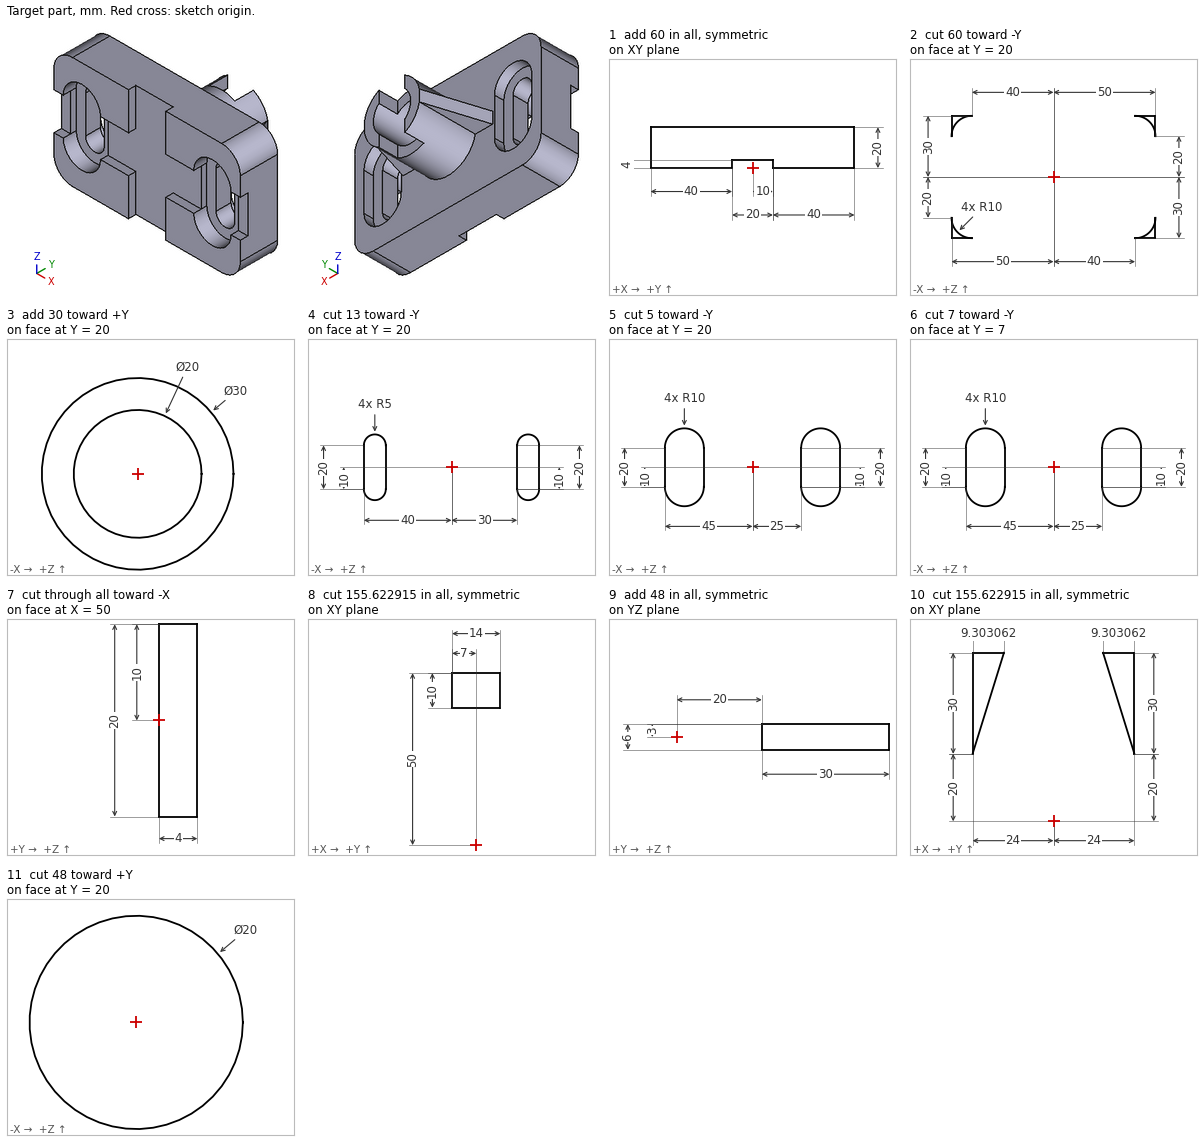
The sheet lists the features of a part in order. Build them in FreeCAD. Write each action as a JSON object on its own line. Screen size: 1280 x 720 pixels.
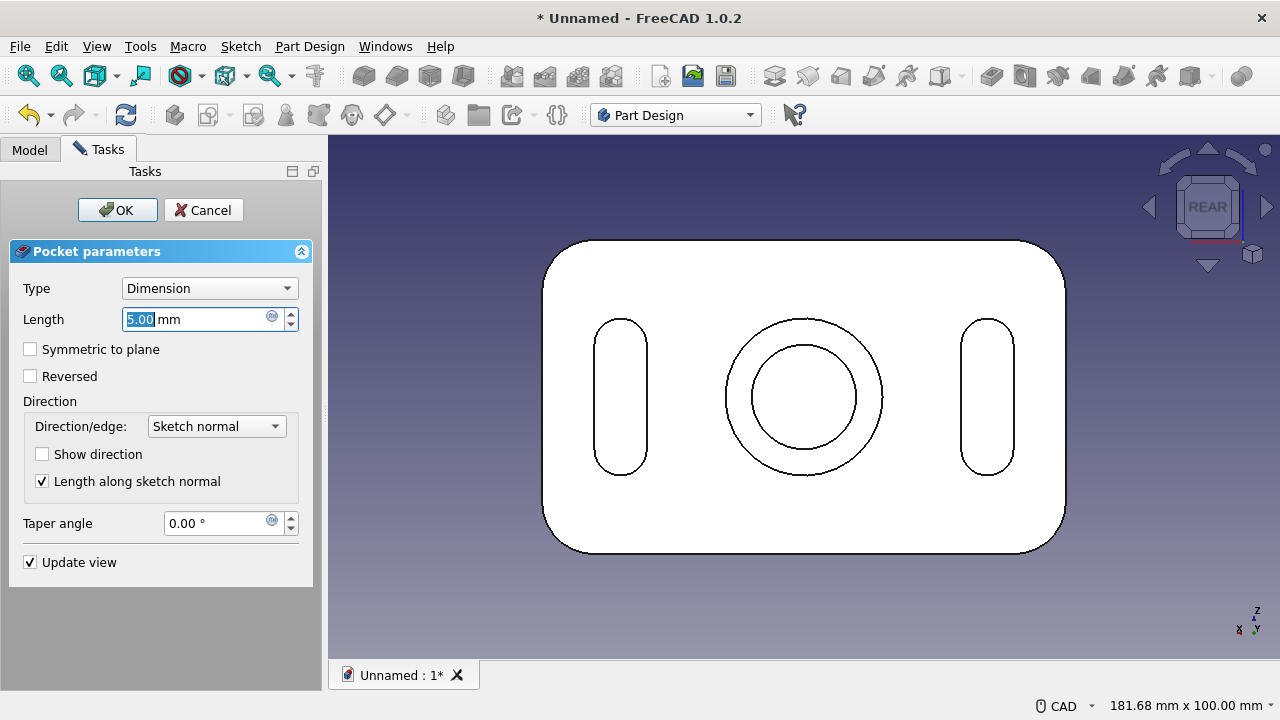
{"action": "type", "text": "13"}
{"action": "key", "text": "Tab"}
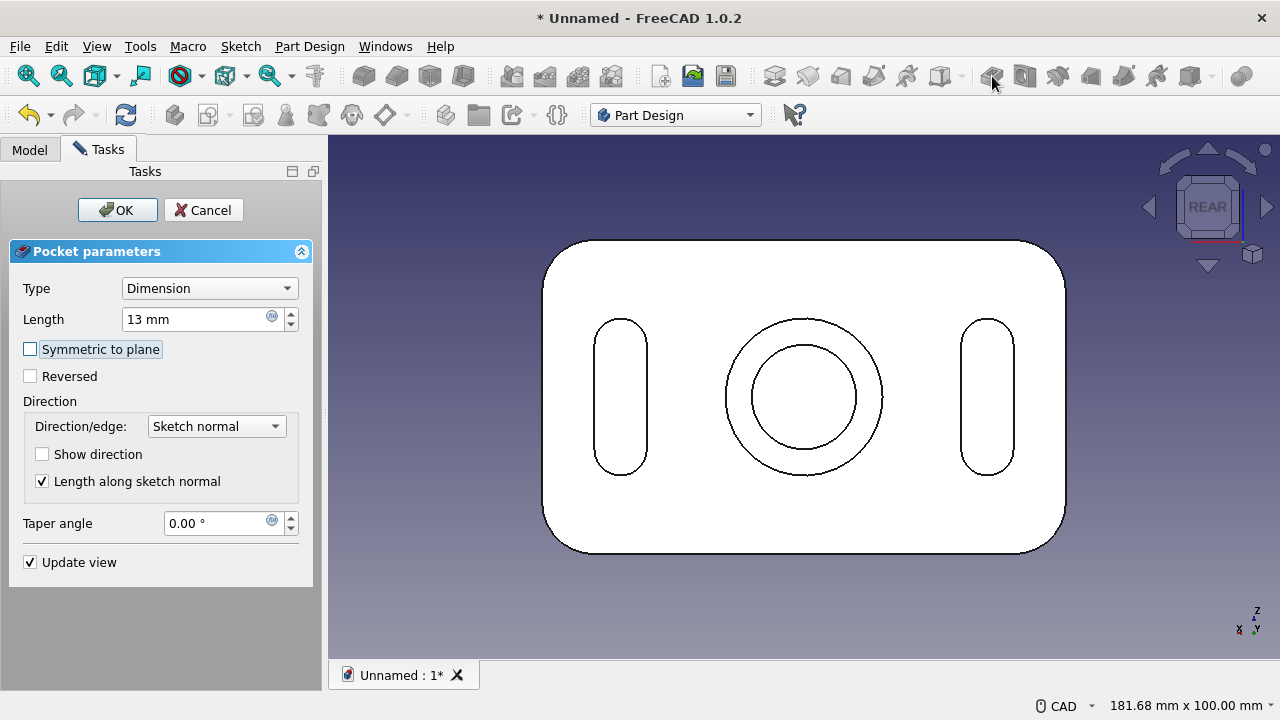
{"action": "left_click", "coordinate": [118, 210]}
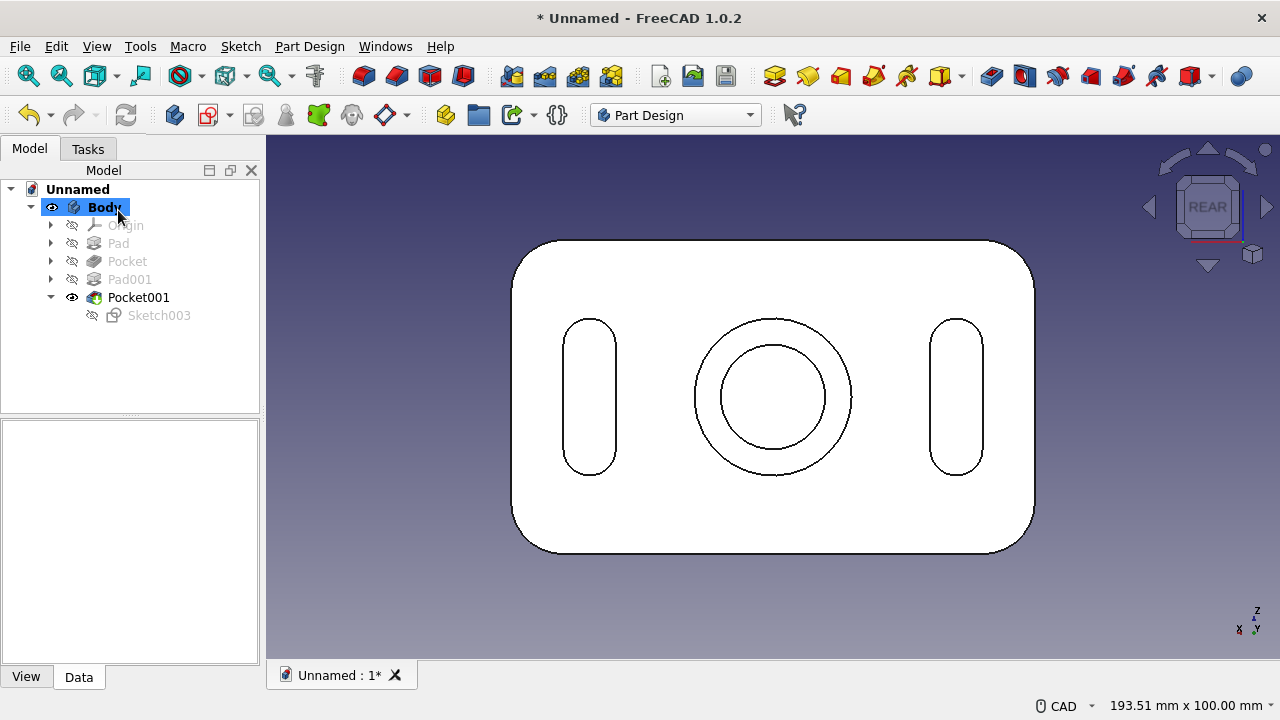
{"action": "left_click", "coordinate": [848, 486]}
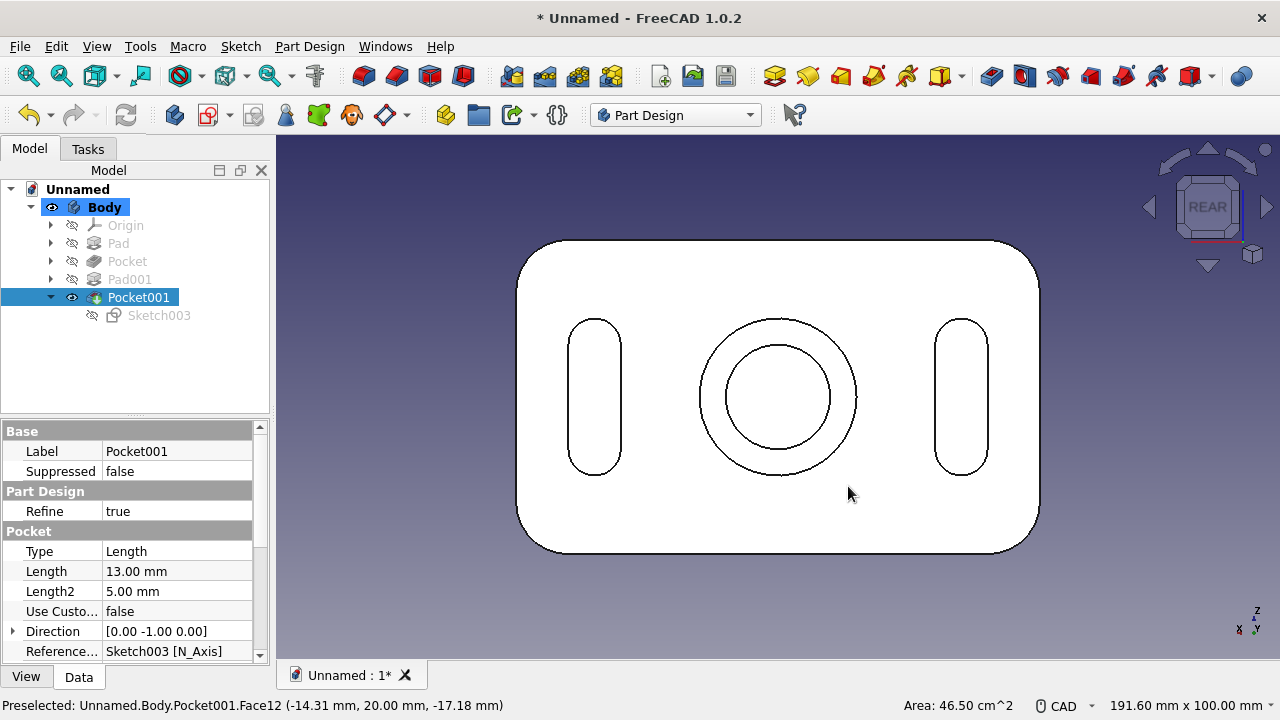
{"action": "left_click", "coordinate": [208, 116]}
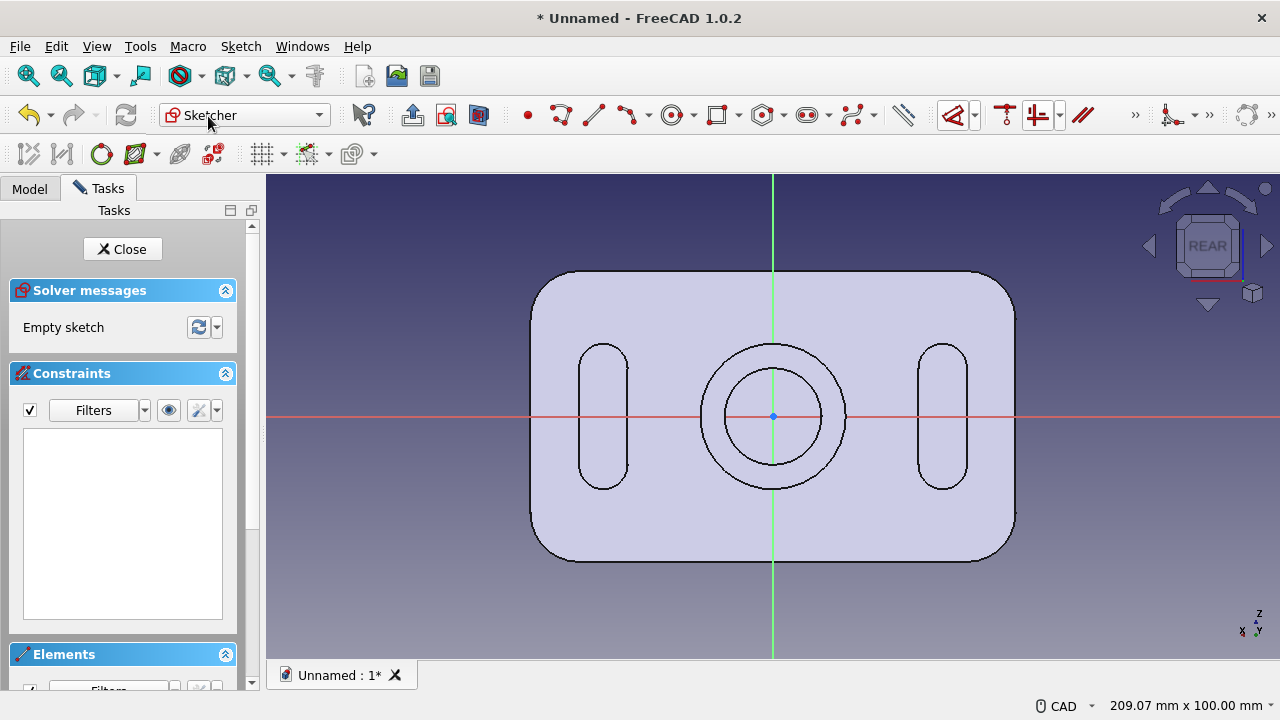
{"action": "key", "text": "g s"}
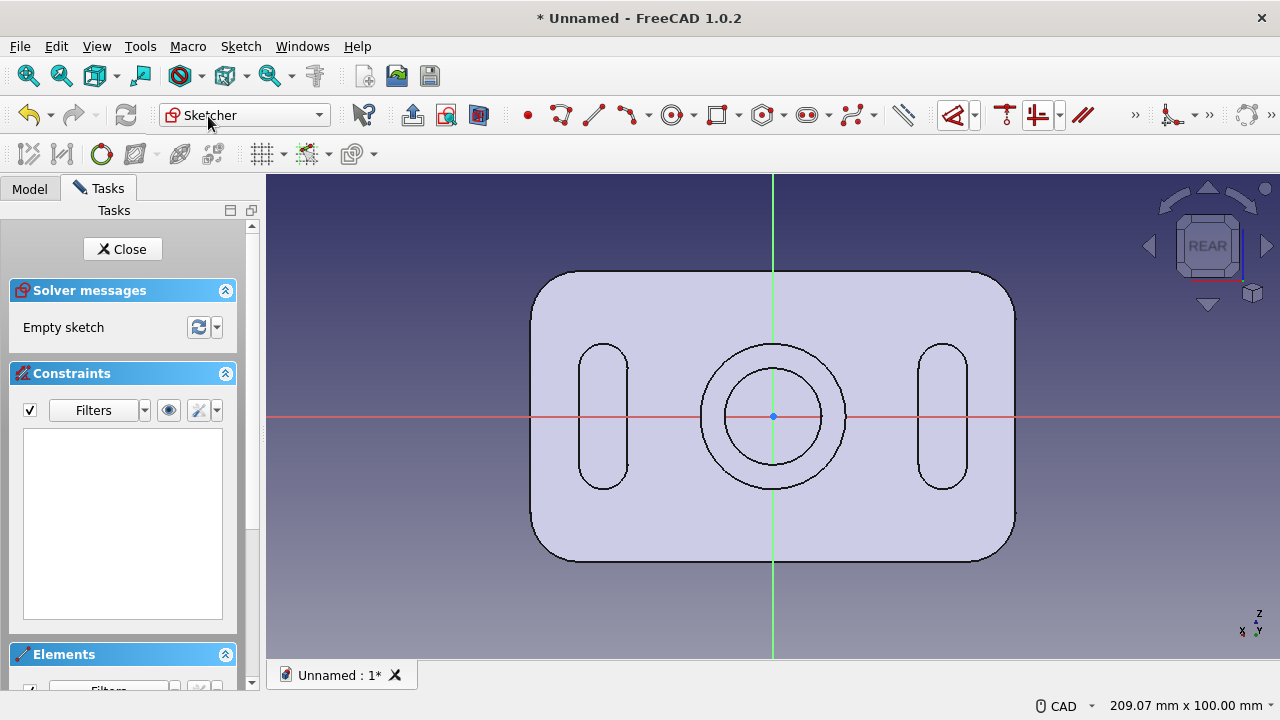
{"action": "left_click", "coordinate": [603, 465]}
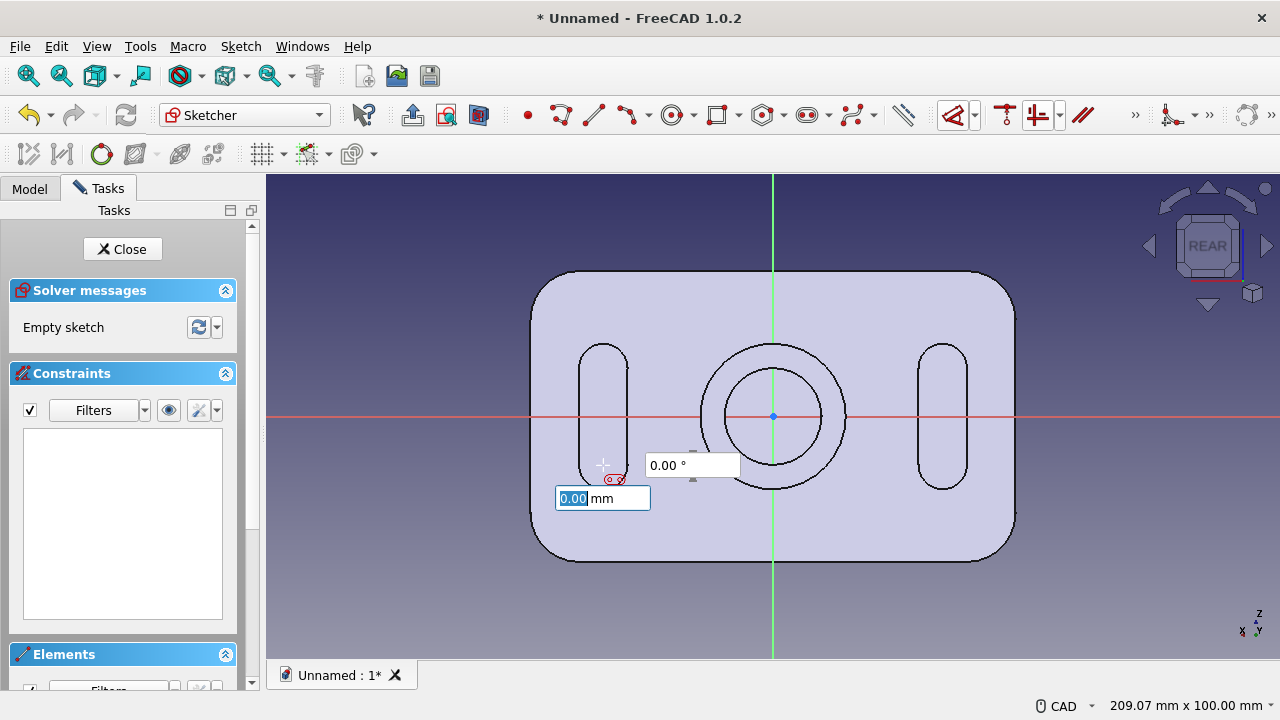
{"action": "left_click", "coordinate": [603, 368]}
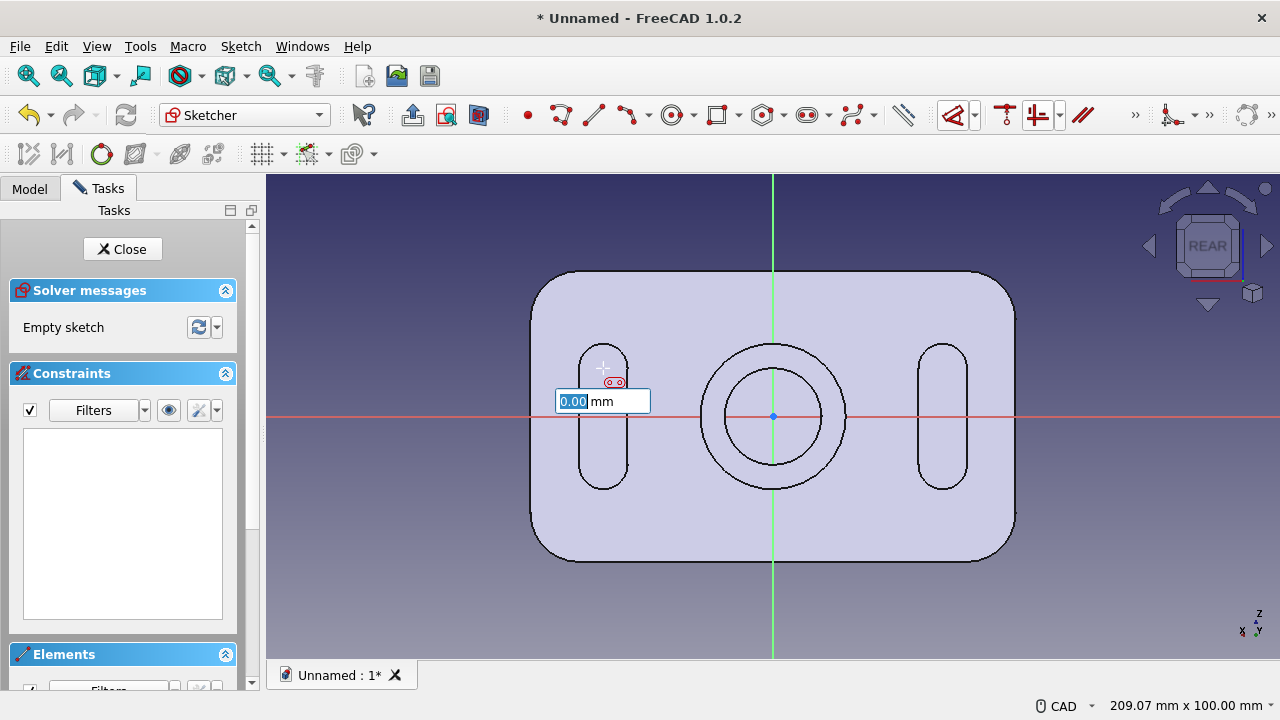
{"action": "left_click", "coordinate": [652, 431]}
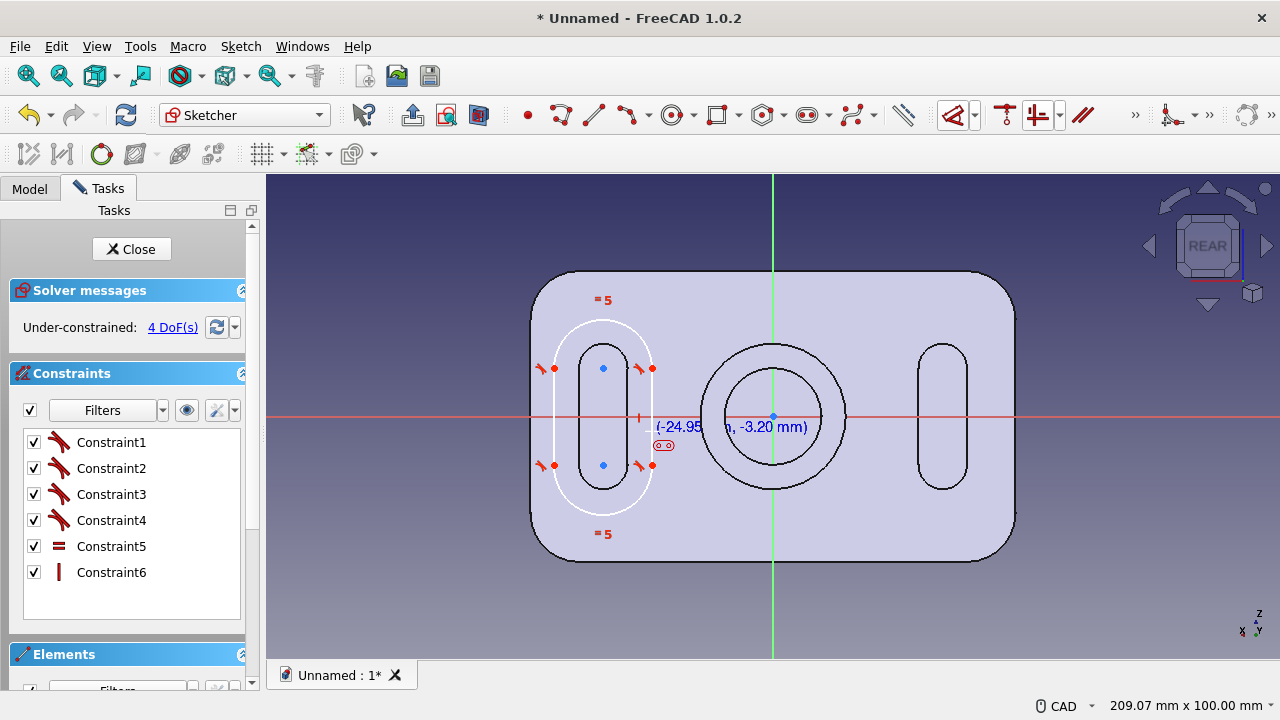
{"action": "left_click", "coordinate": [943, 465]}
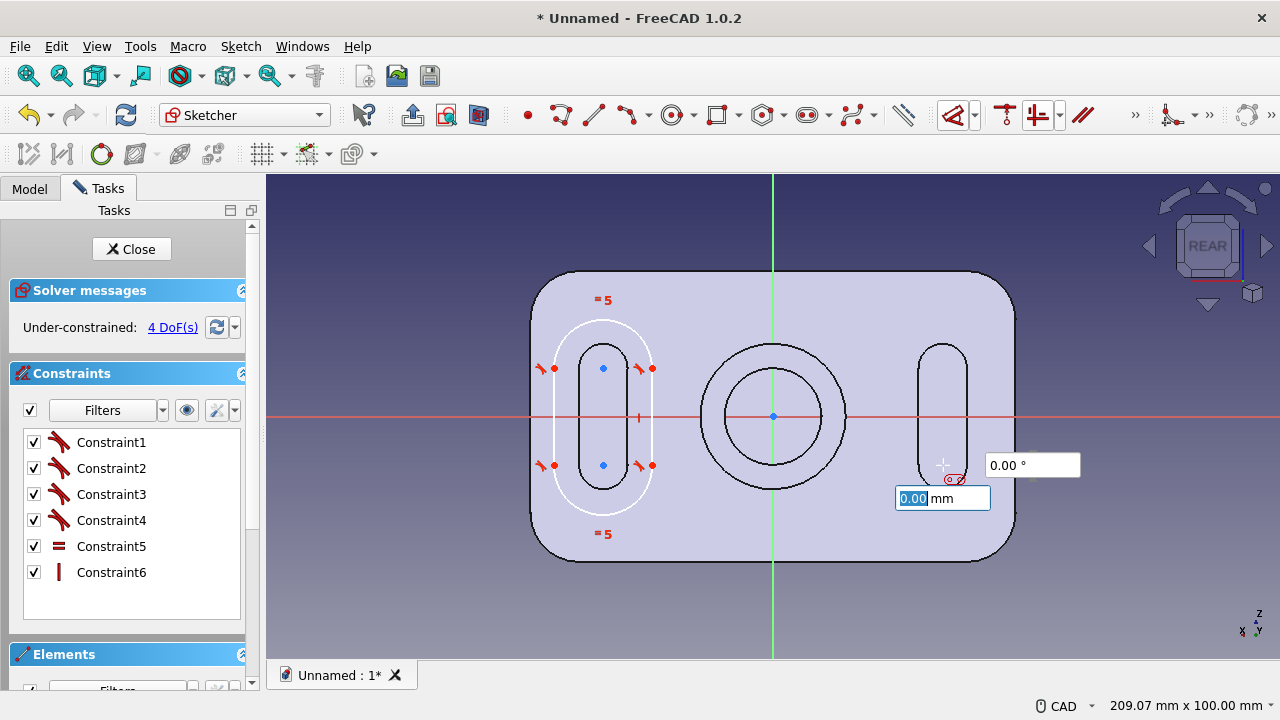
{"action": "left_click", "coordinate": [943, 368]}